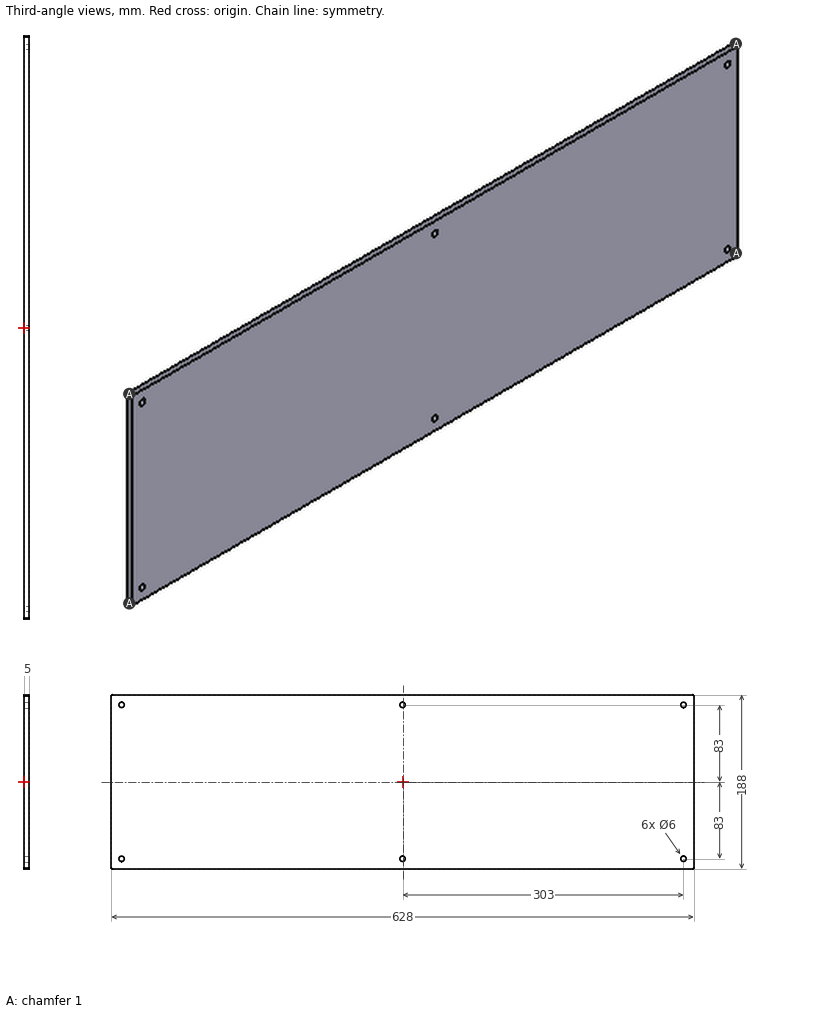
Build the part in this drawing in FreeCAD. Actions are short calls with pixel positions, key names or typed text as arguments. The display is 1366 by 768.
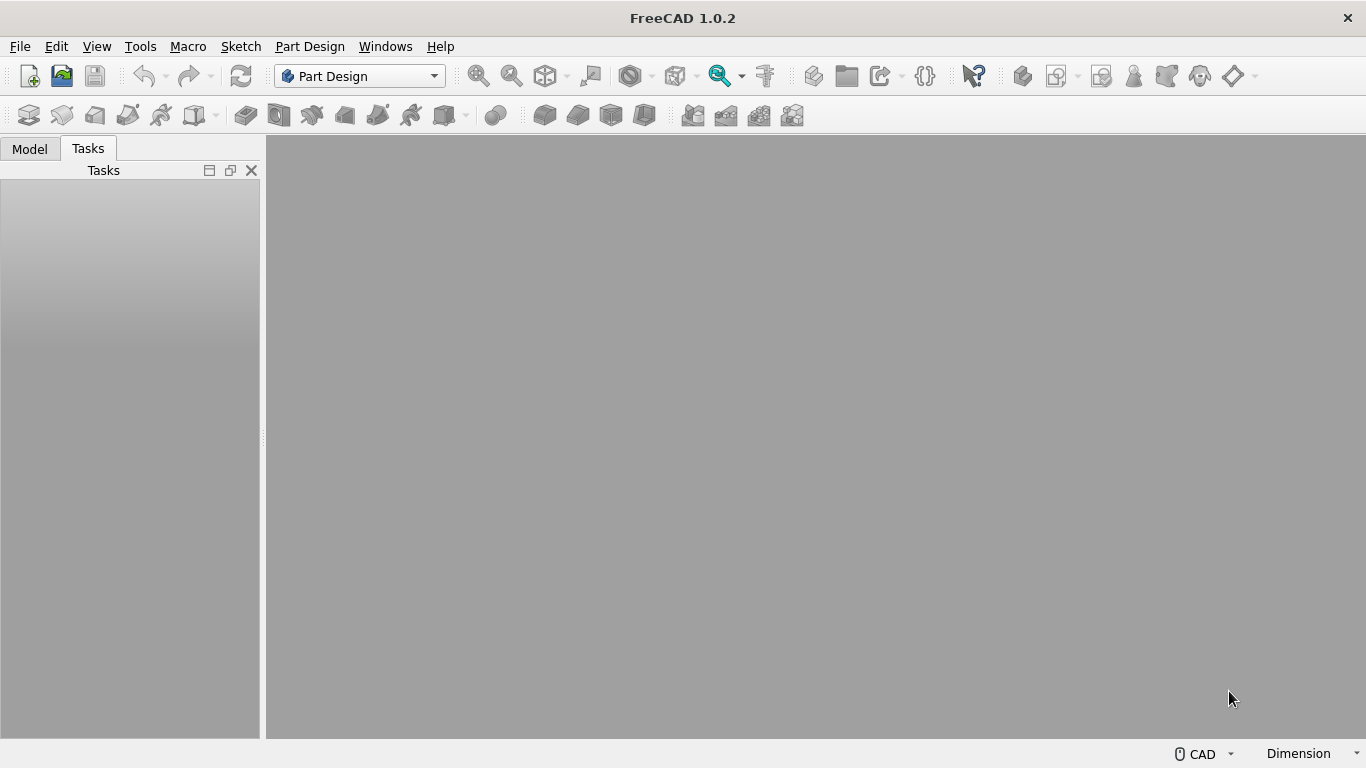
key(ctrl+n)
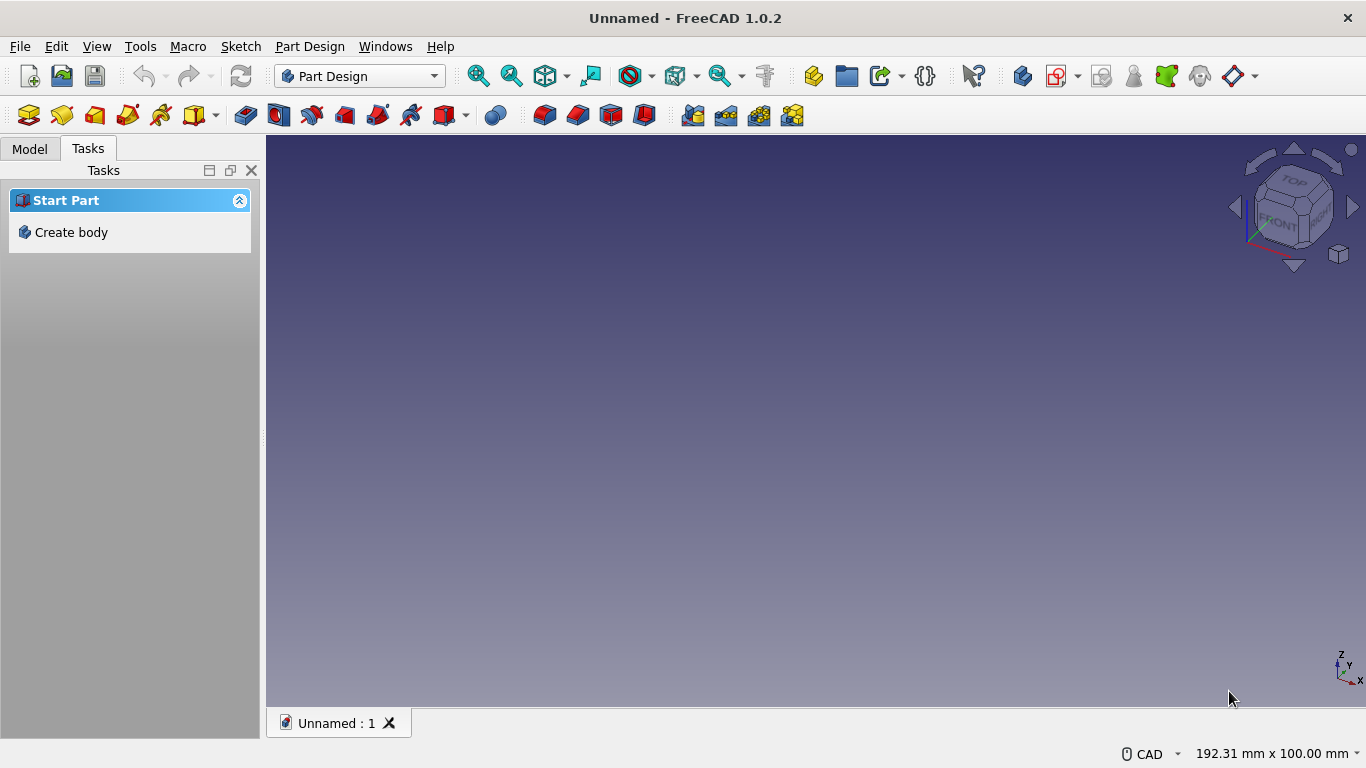
click(1056, 76)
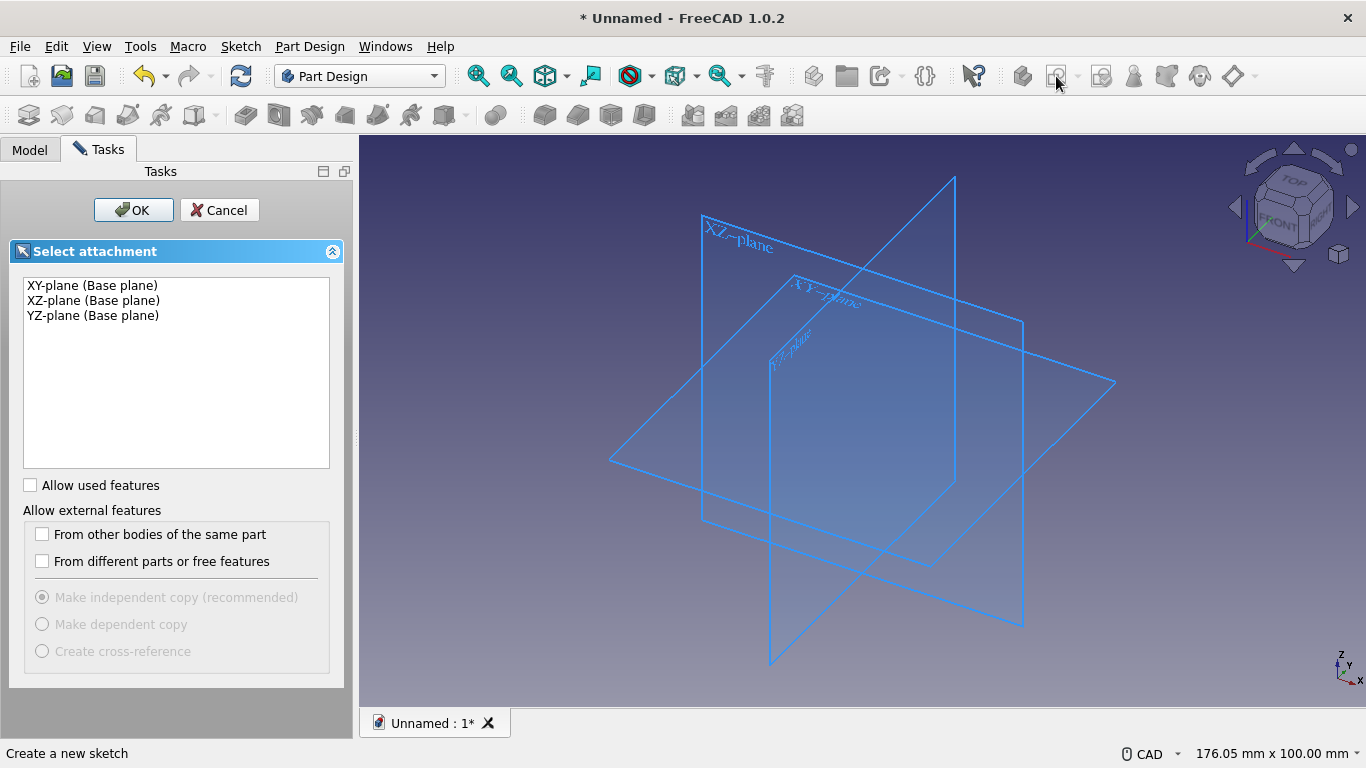
click(84, 316)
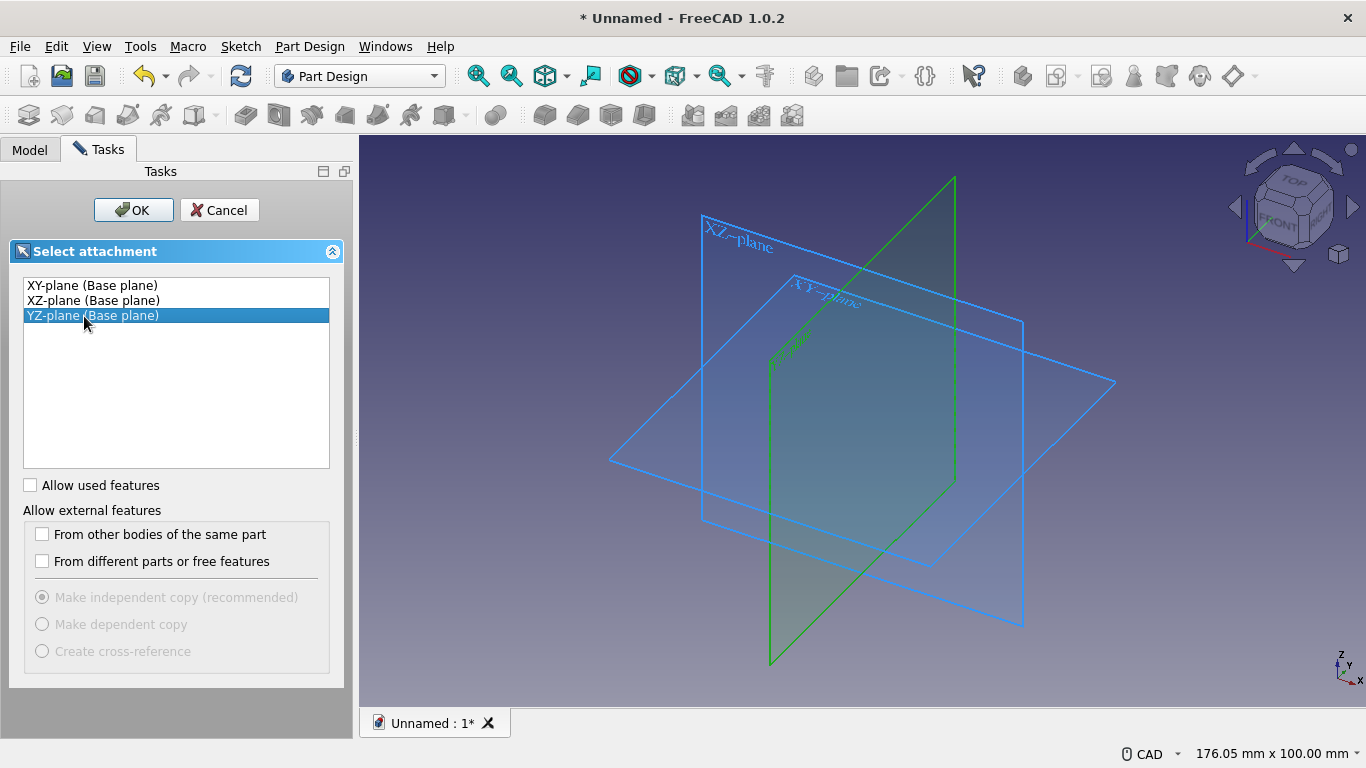
click(134, 210)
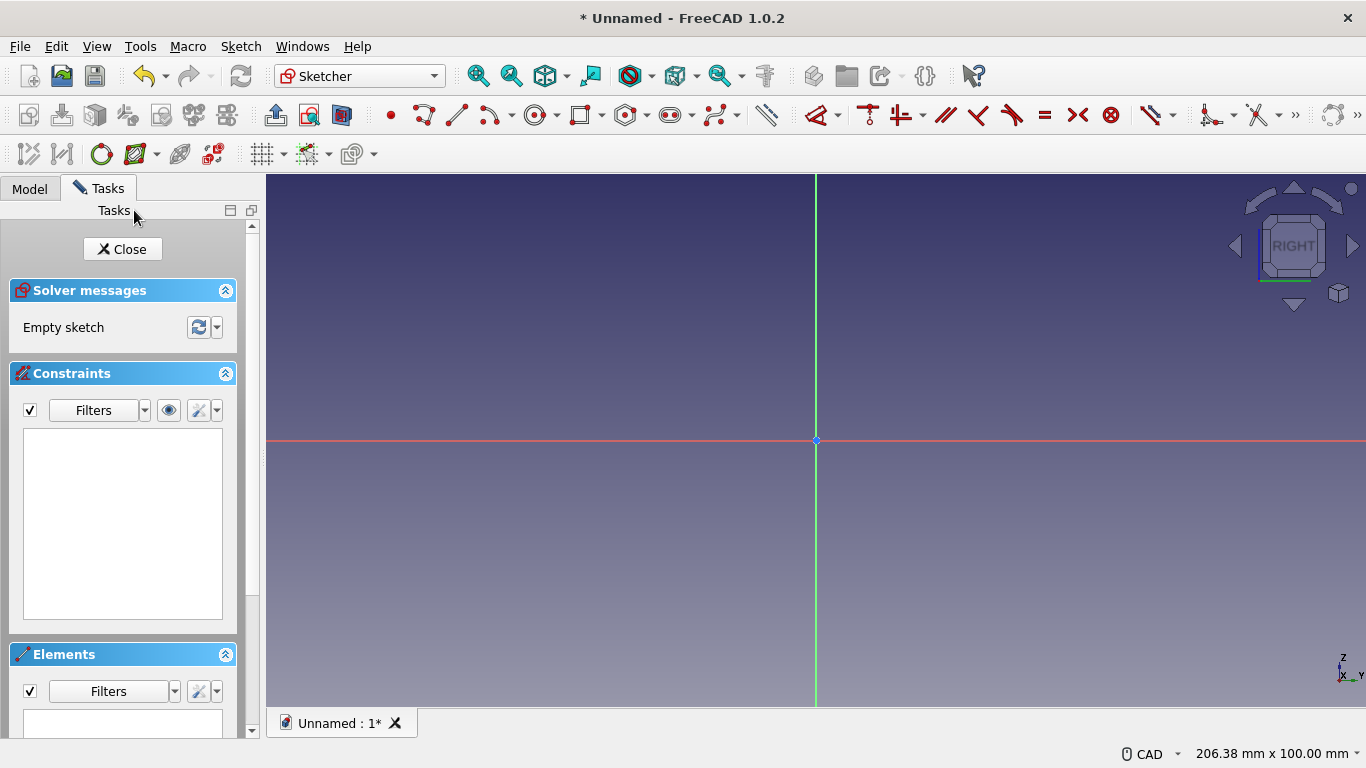
scroll(730, 440, down, 8)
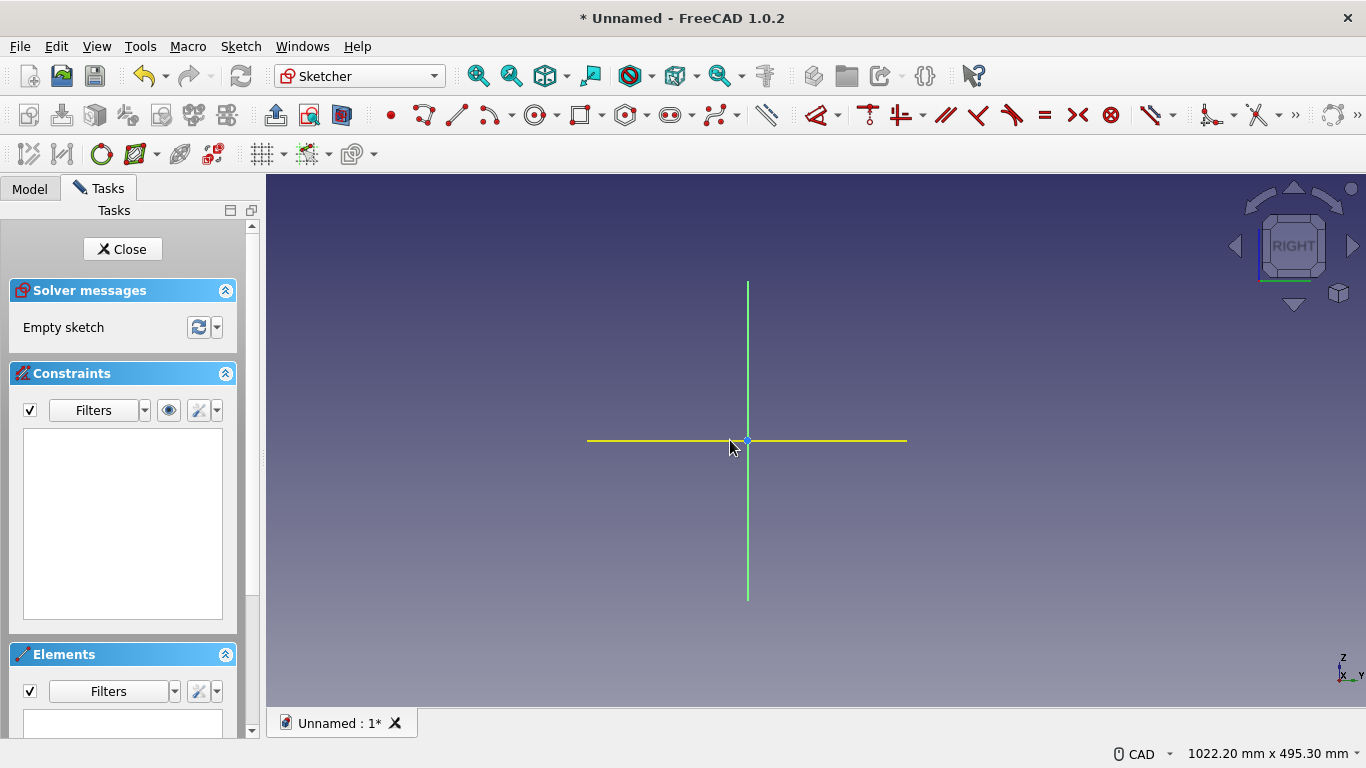
key(g)
key(v)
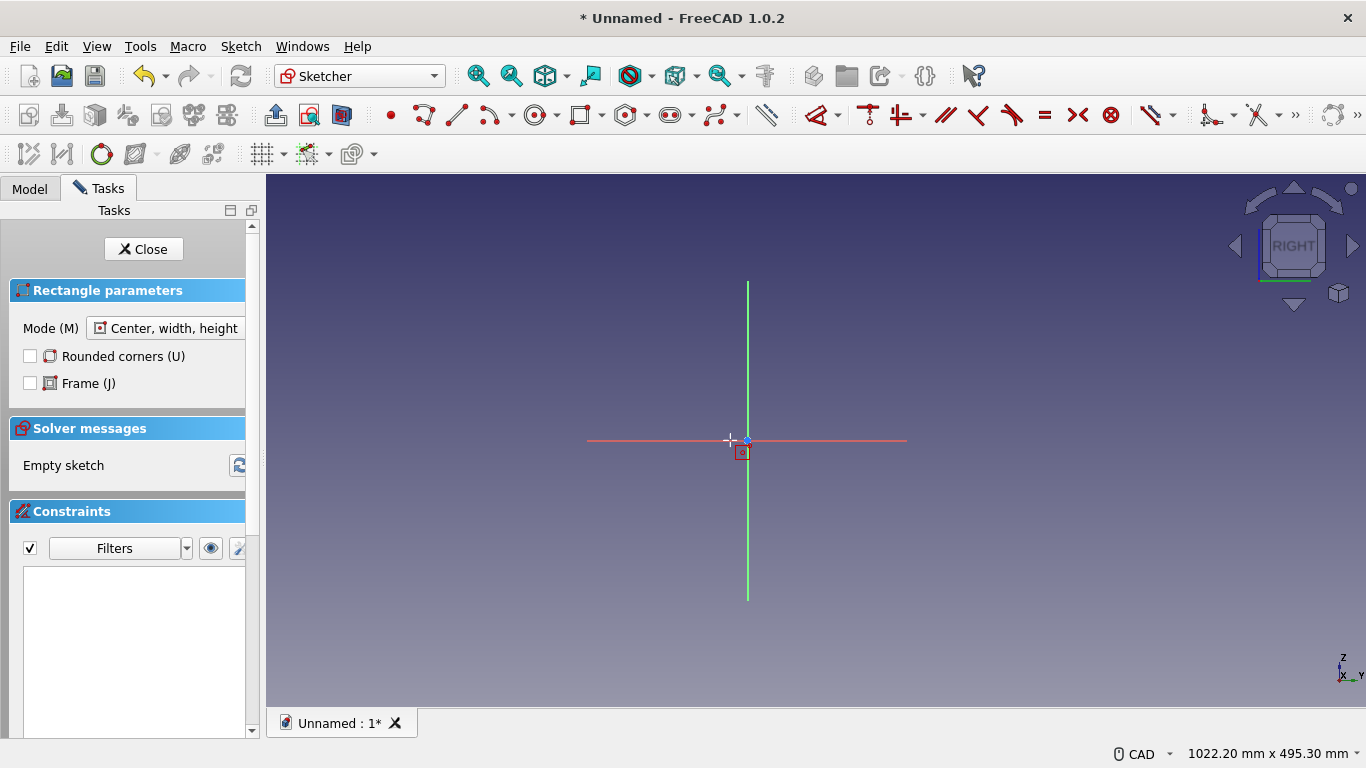
click(748, 440)
move(1086, 339)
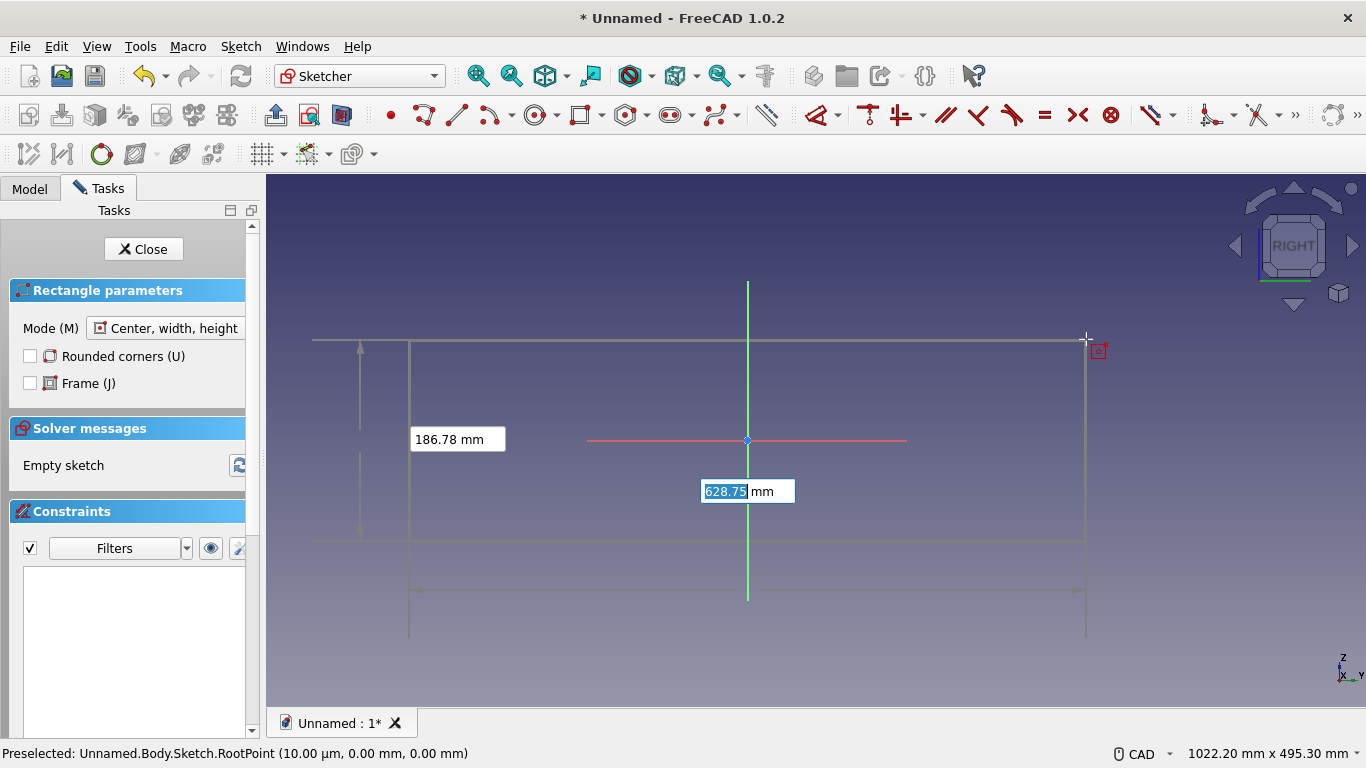
text(628)
key(Tab)
text(188)
key(Return)
key(Escape)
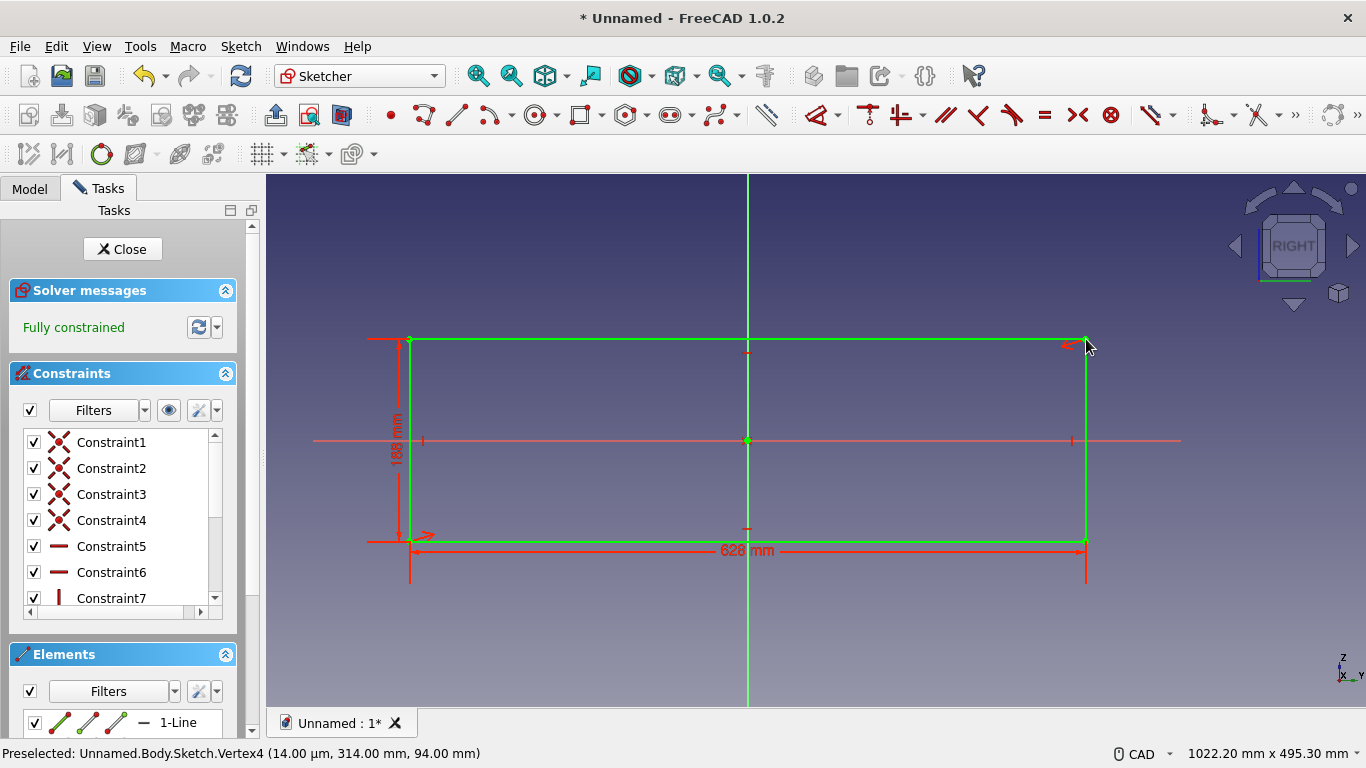
click(123, 249)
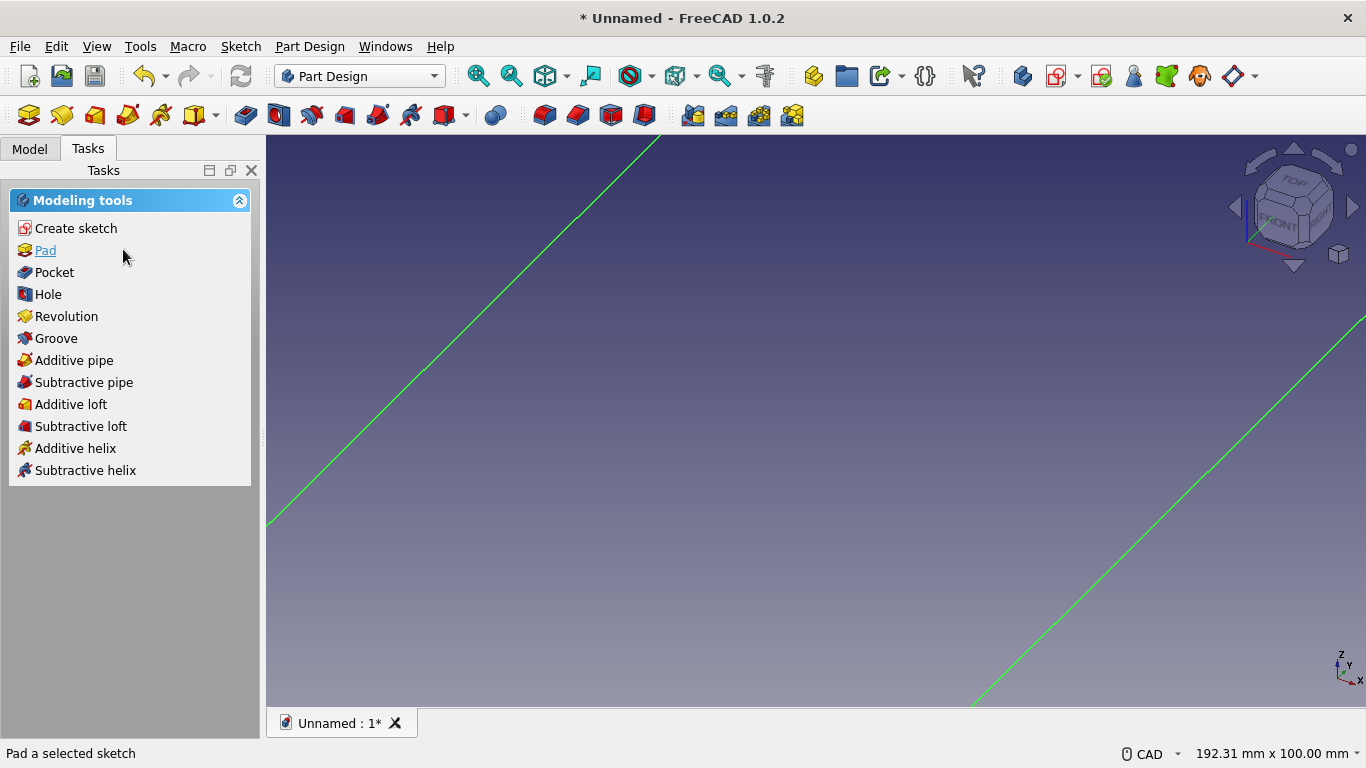
click(29, 116)